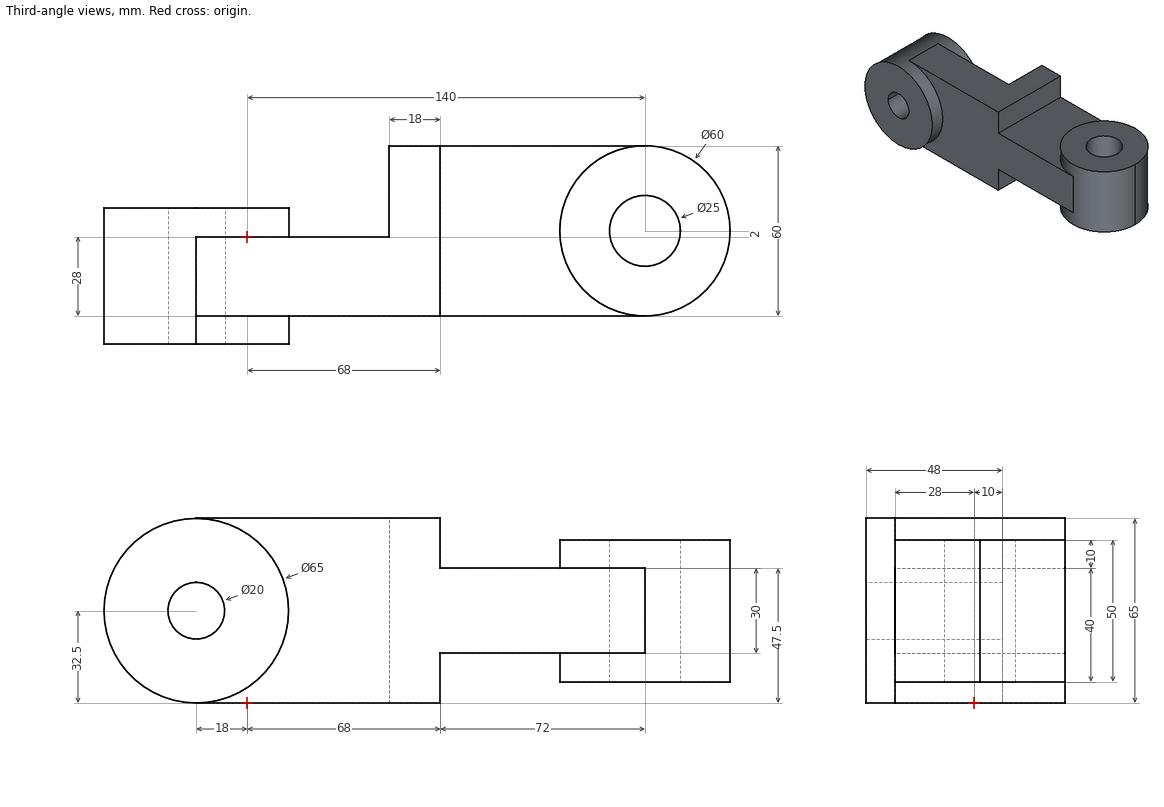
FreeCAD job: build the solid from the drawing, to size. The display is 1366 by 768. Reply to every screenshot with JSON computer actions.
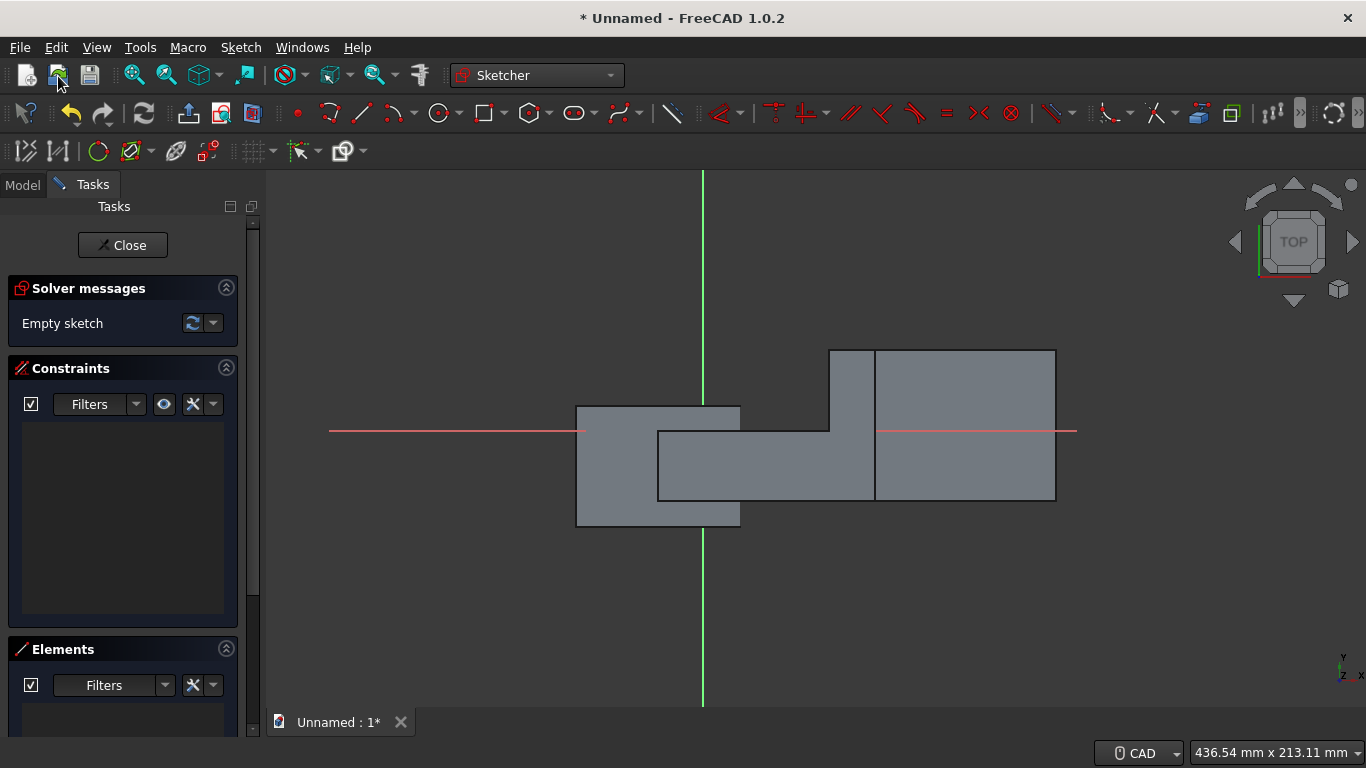
{"action": "scroll", "coordinate": [1201, 416], "scroll_direction": "up", "scroll_amount": 4}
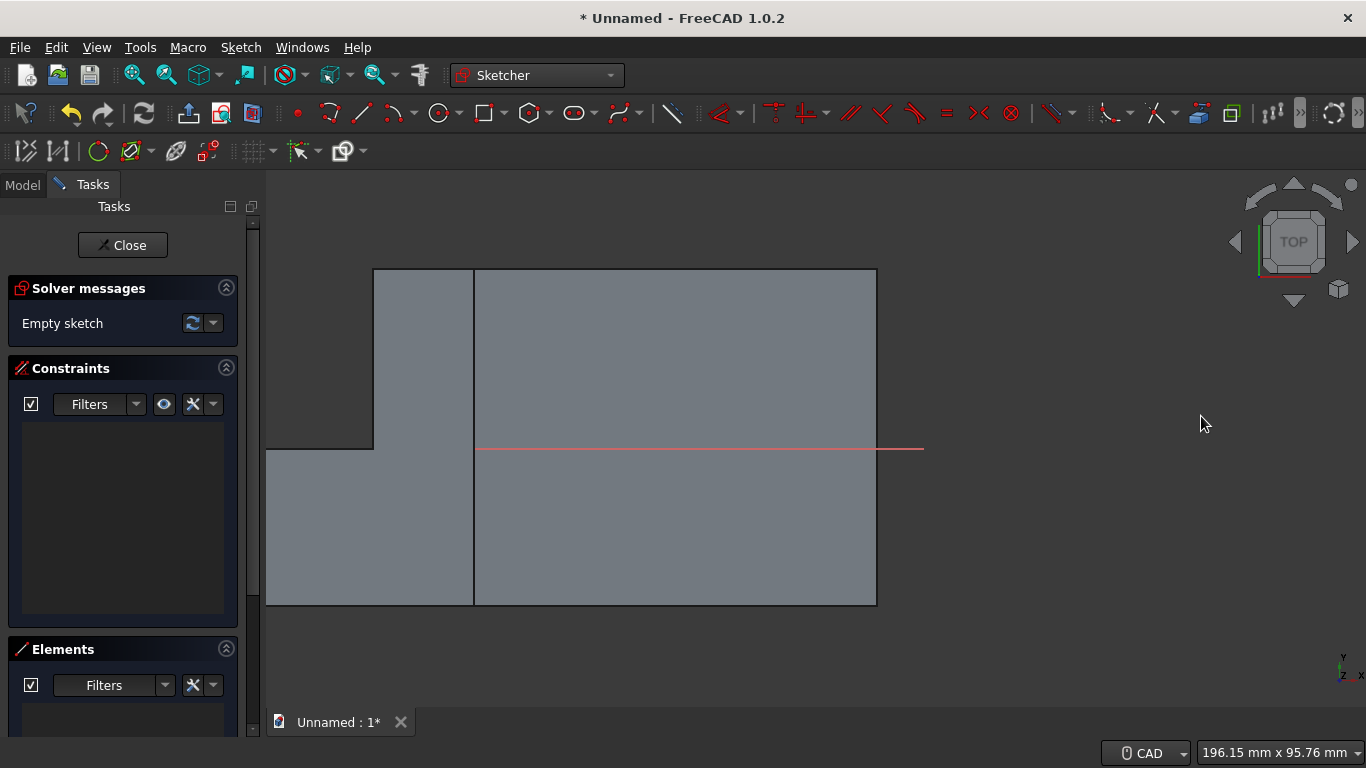
{"action": "left_click", "coordinate": [440, 114]}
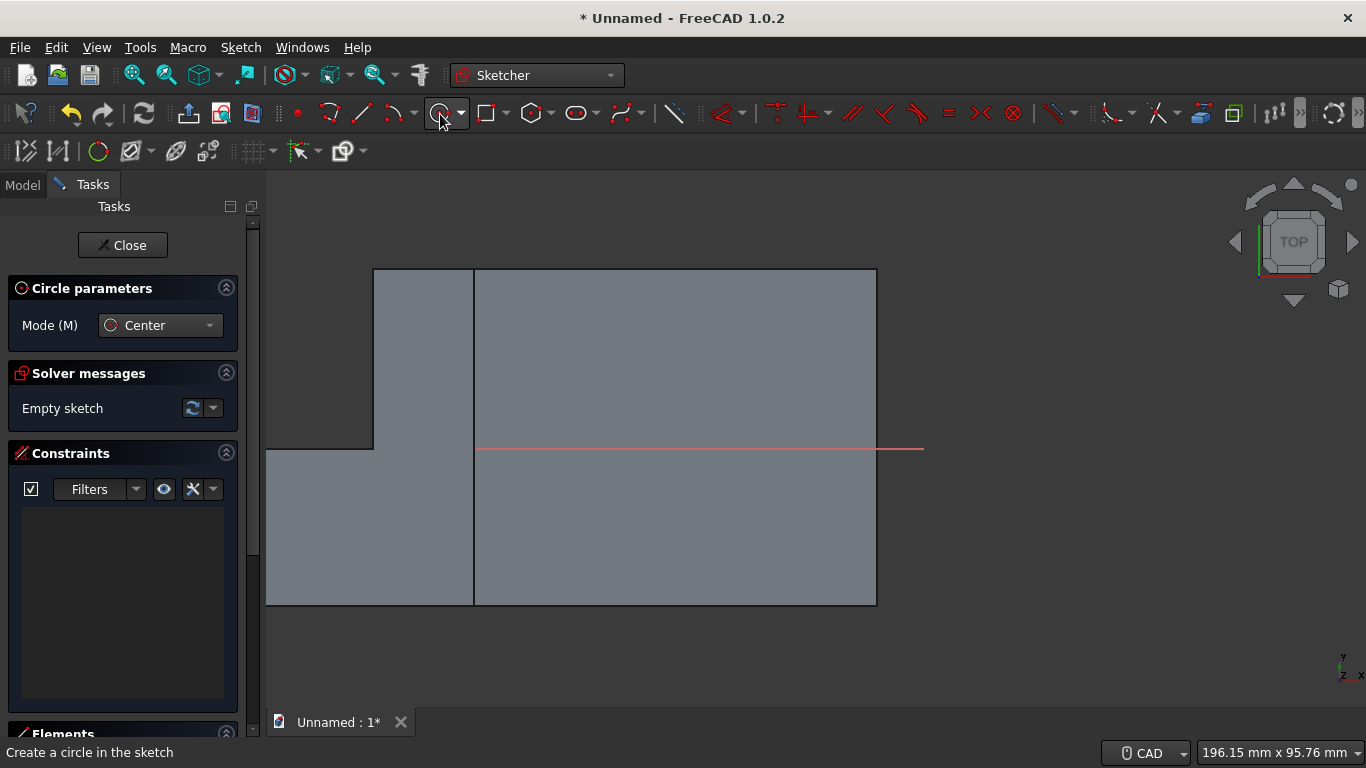
{"action": "scroll", "coordinate": [877, 437], "scroll_direction": "up", "scroll_amount": 2}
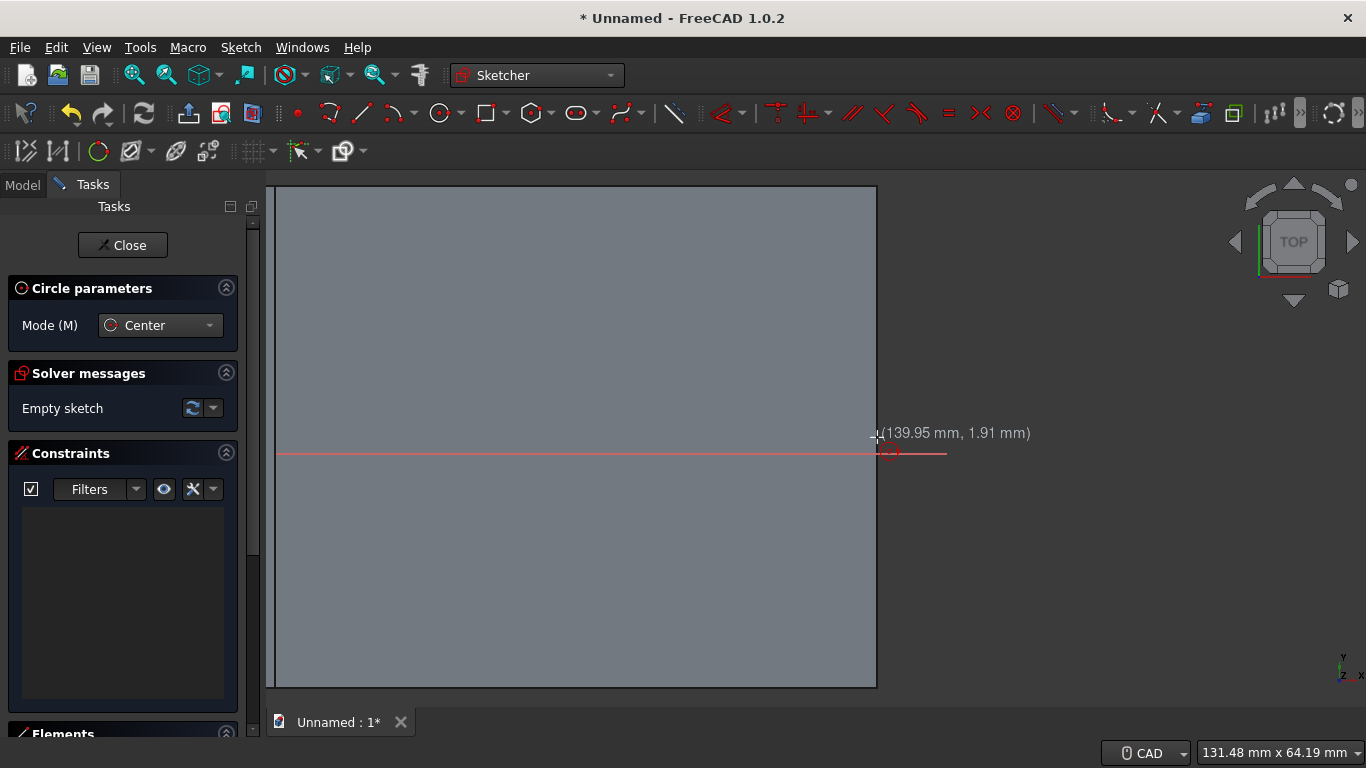
{"action": "left_click", "coordinate": [877, 437]}
{"action": "left_click", "coordinate": [1055, 260]}
{"action": "key", "text": "Escape"}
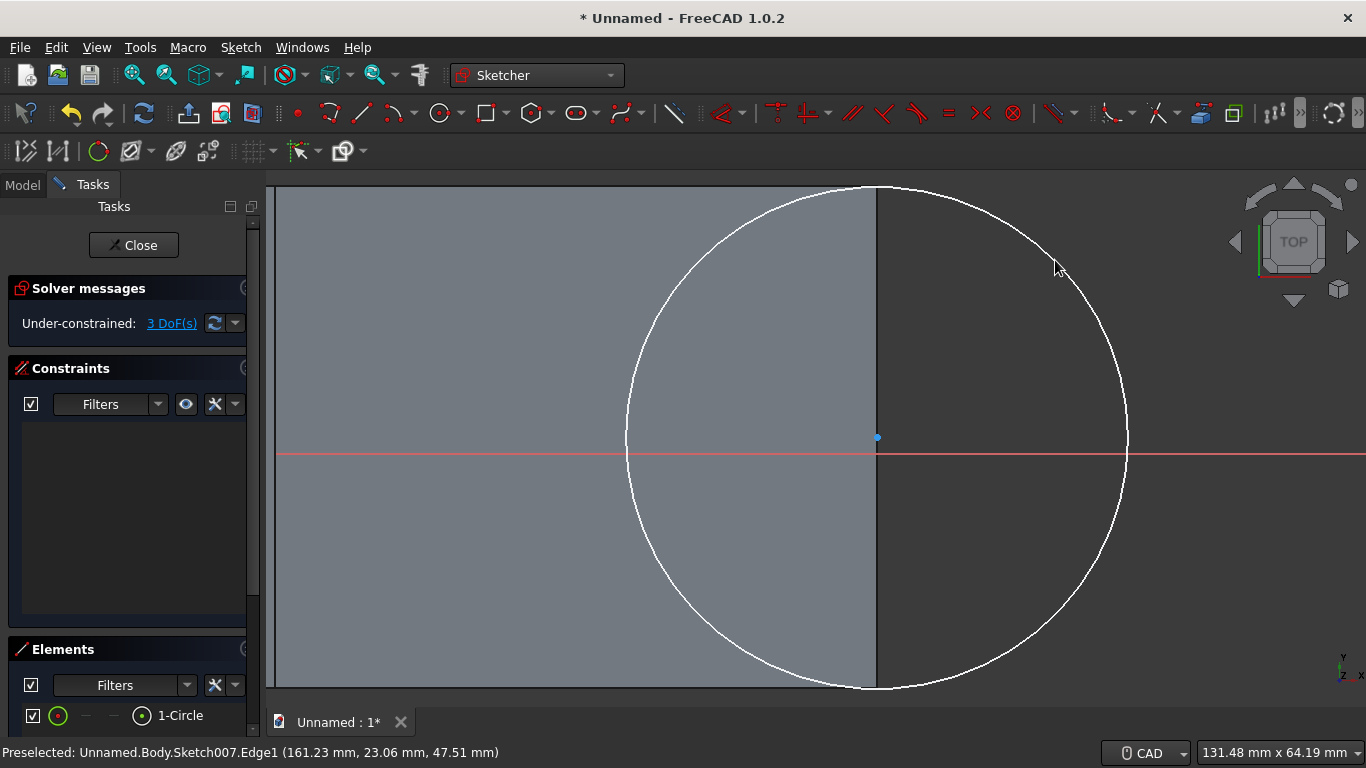
{"action": "key", "text": "d"}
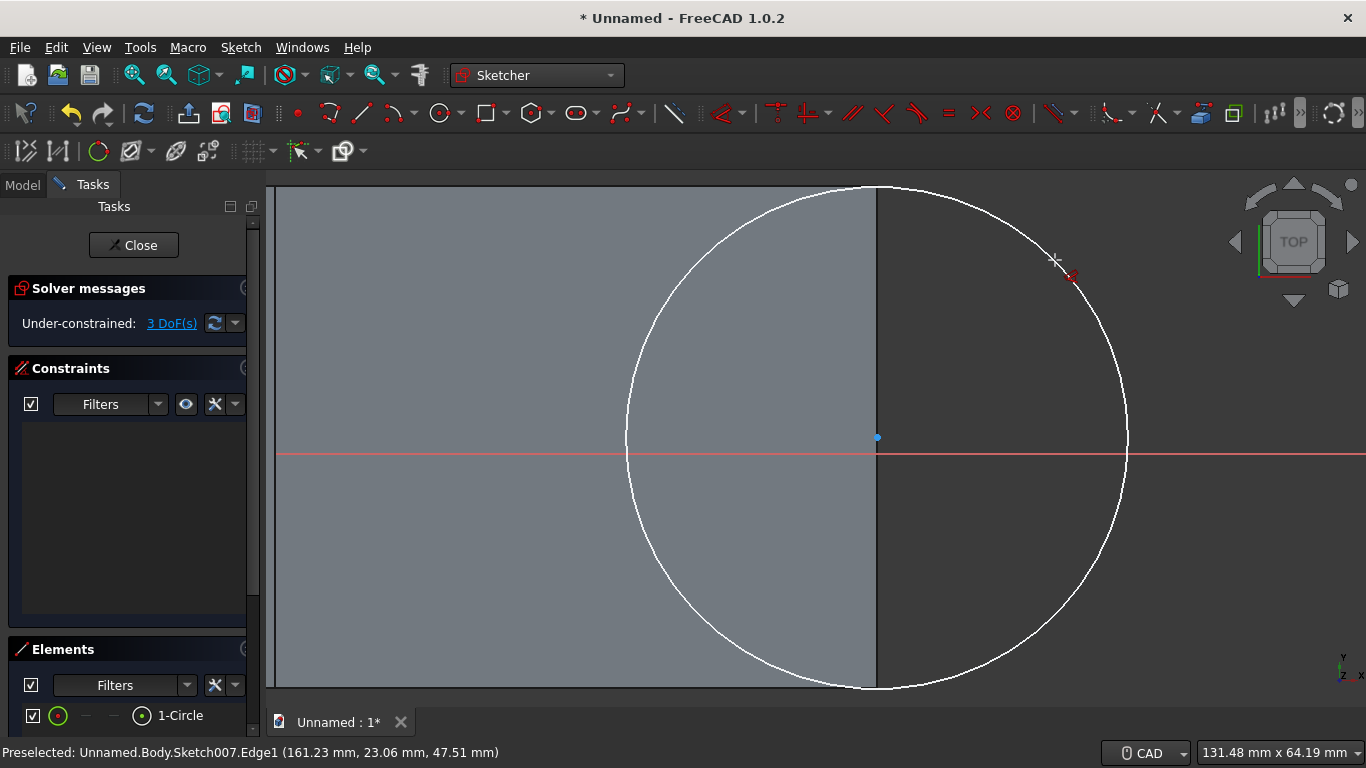
{"action": "left_click", "coordinate": [1054, 260]}
{"action": "left_click", "coordinate": [1077, 237]}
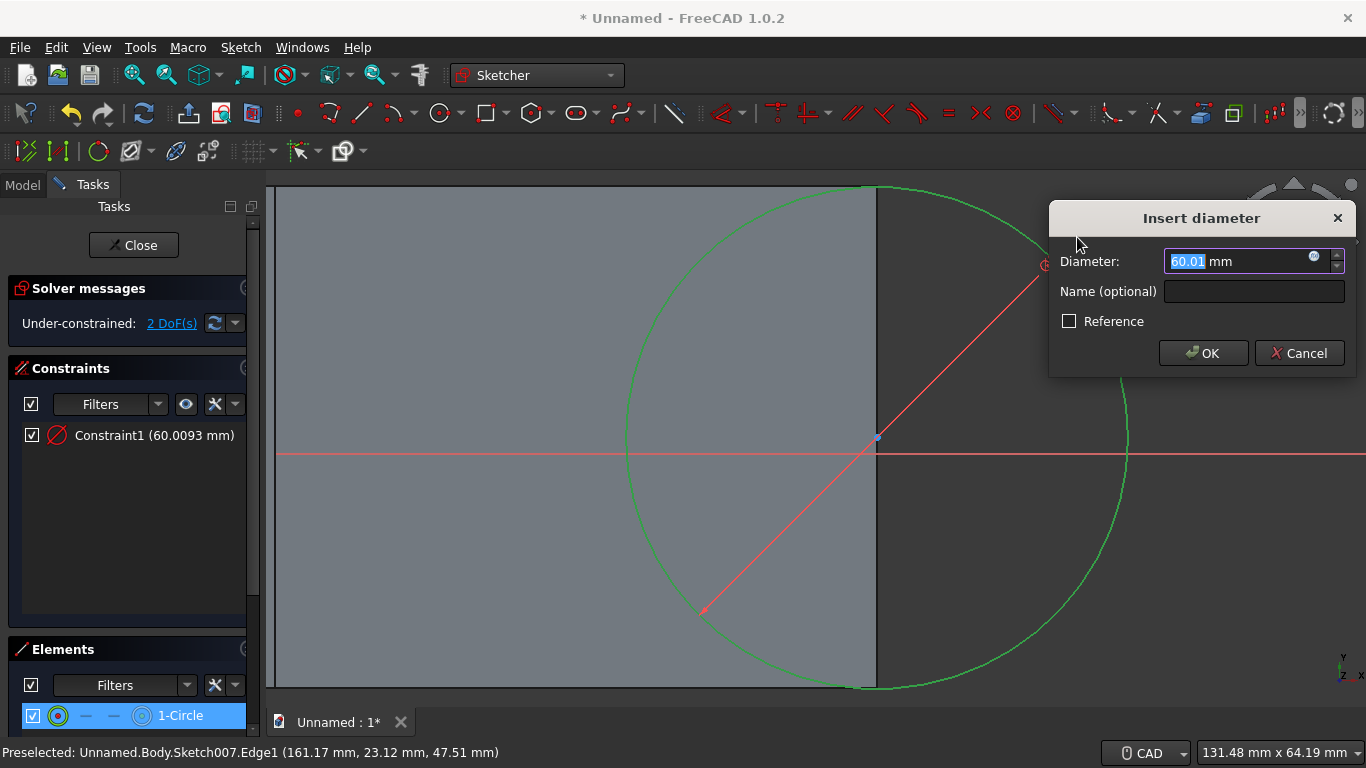
{"action": "type", "text": "60"}
{"action": "key", "text": "Return"}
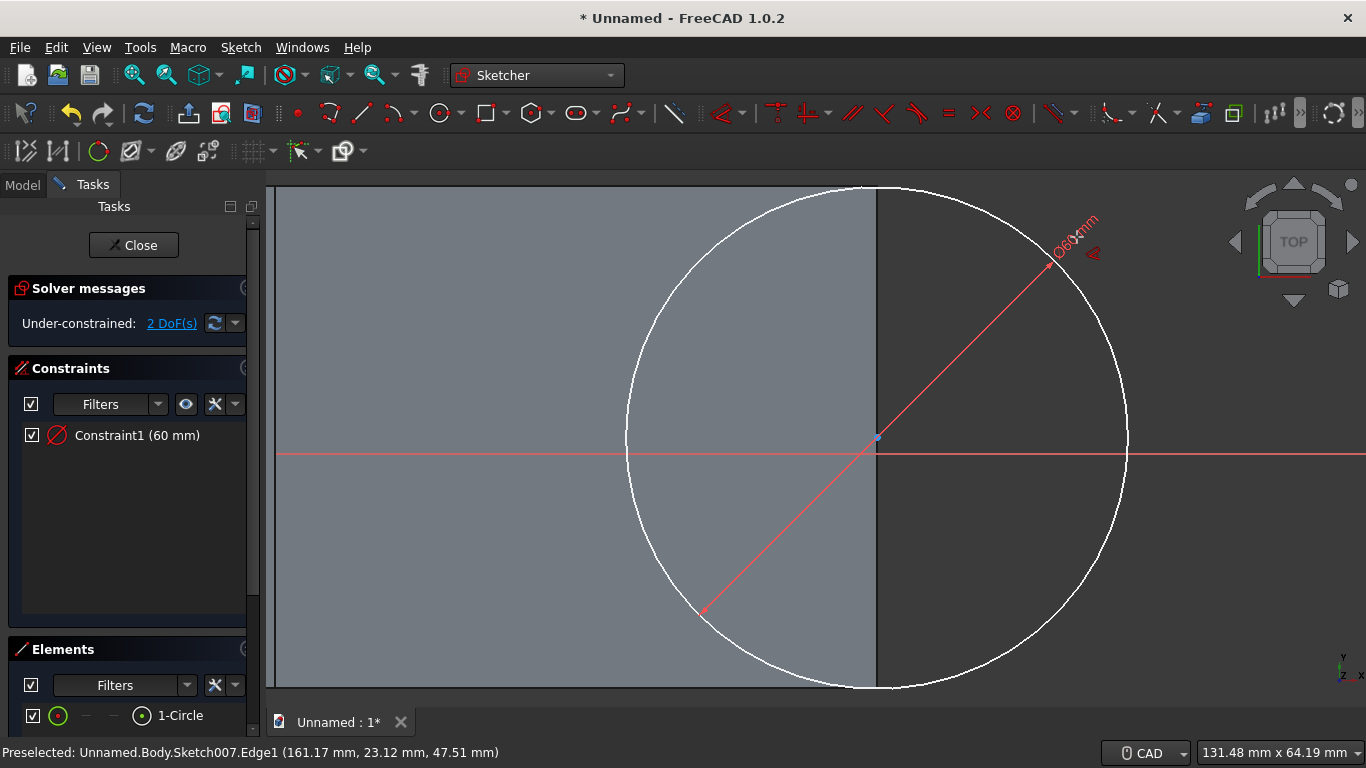
{"action": "scroll", "coordinate": [877, 438], "scroll_direction": "up", "scroll_amount": 5}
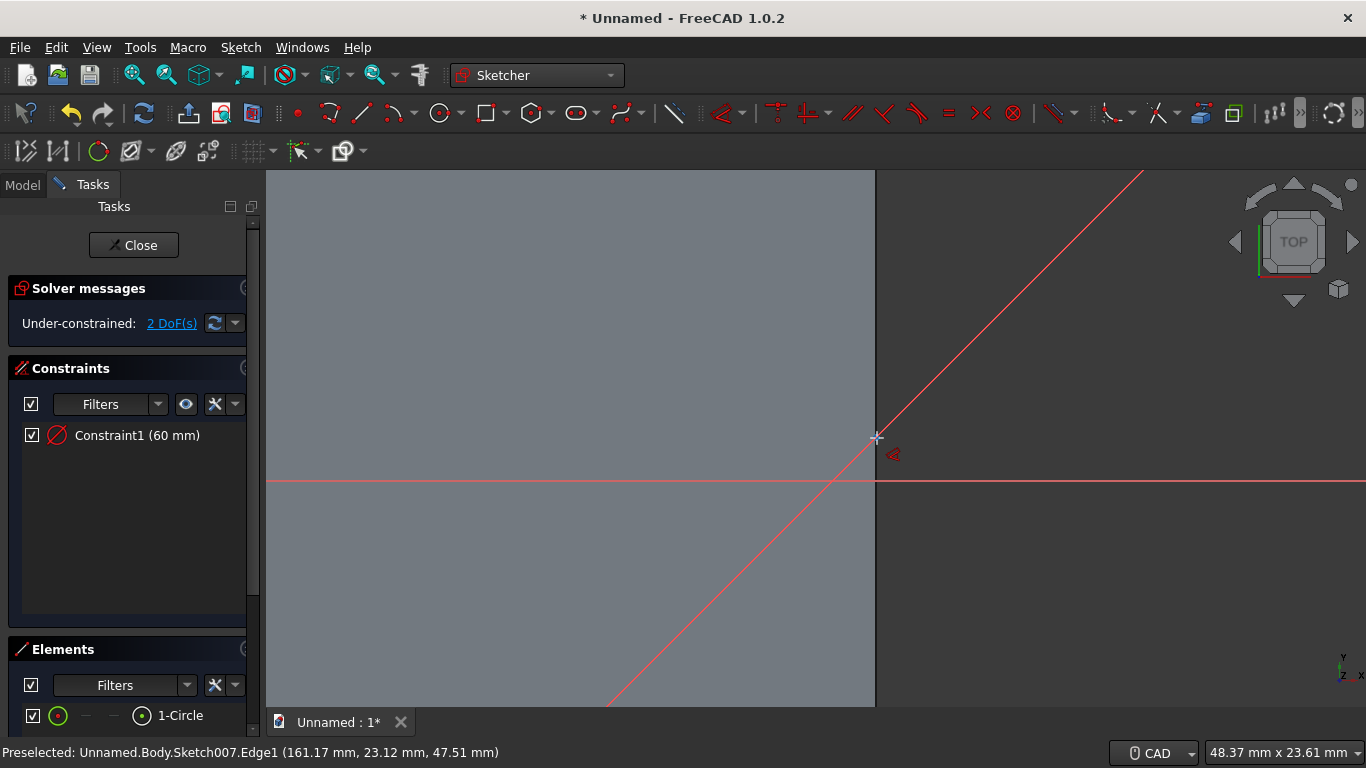
{"action": "left_click", "coordinate": [876, 437]}
{"action": "left_click", "coordinate": [910, 459]}